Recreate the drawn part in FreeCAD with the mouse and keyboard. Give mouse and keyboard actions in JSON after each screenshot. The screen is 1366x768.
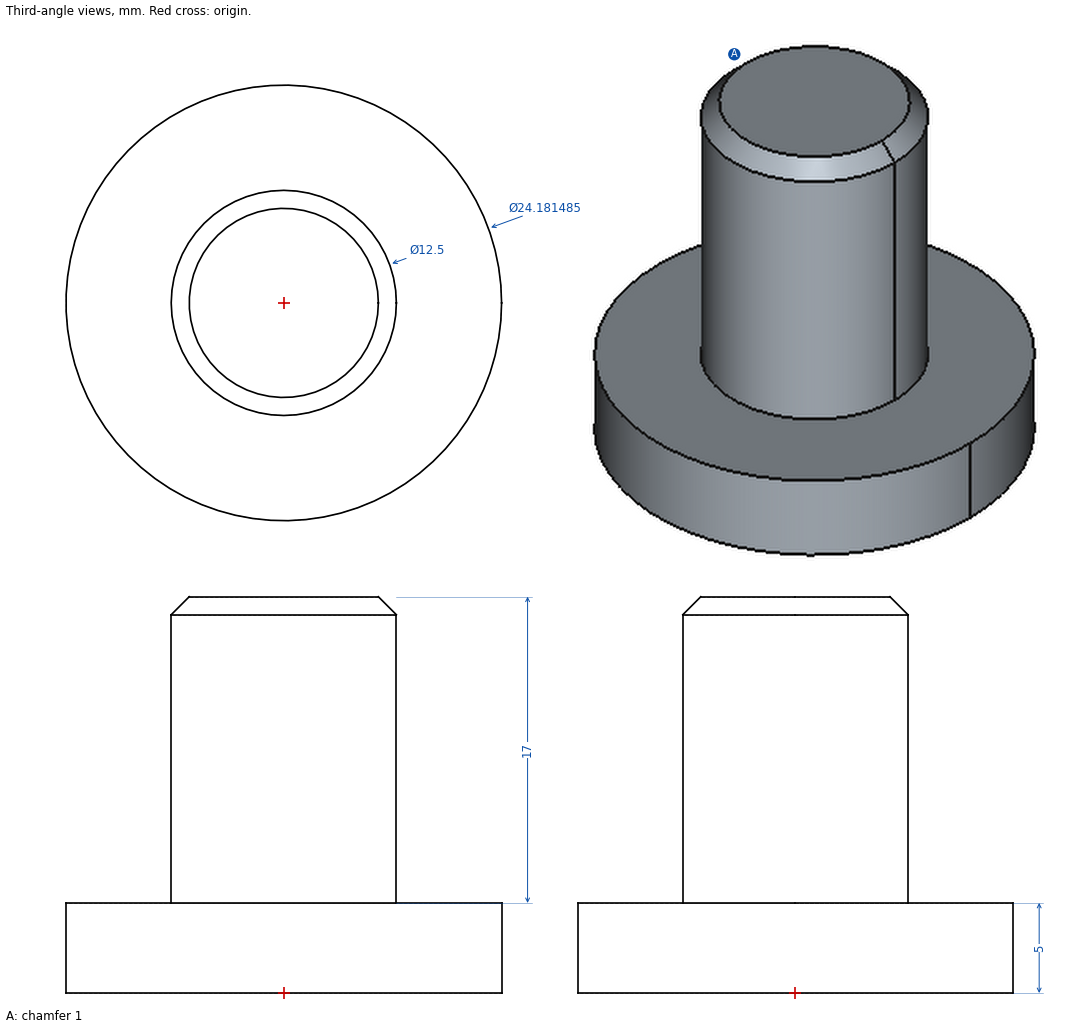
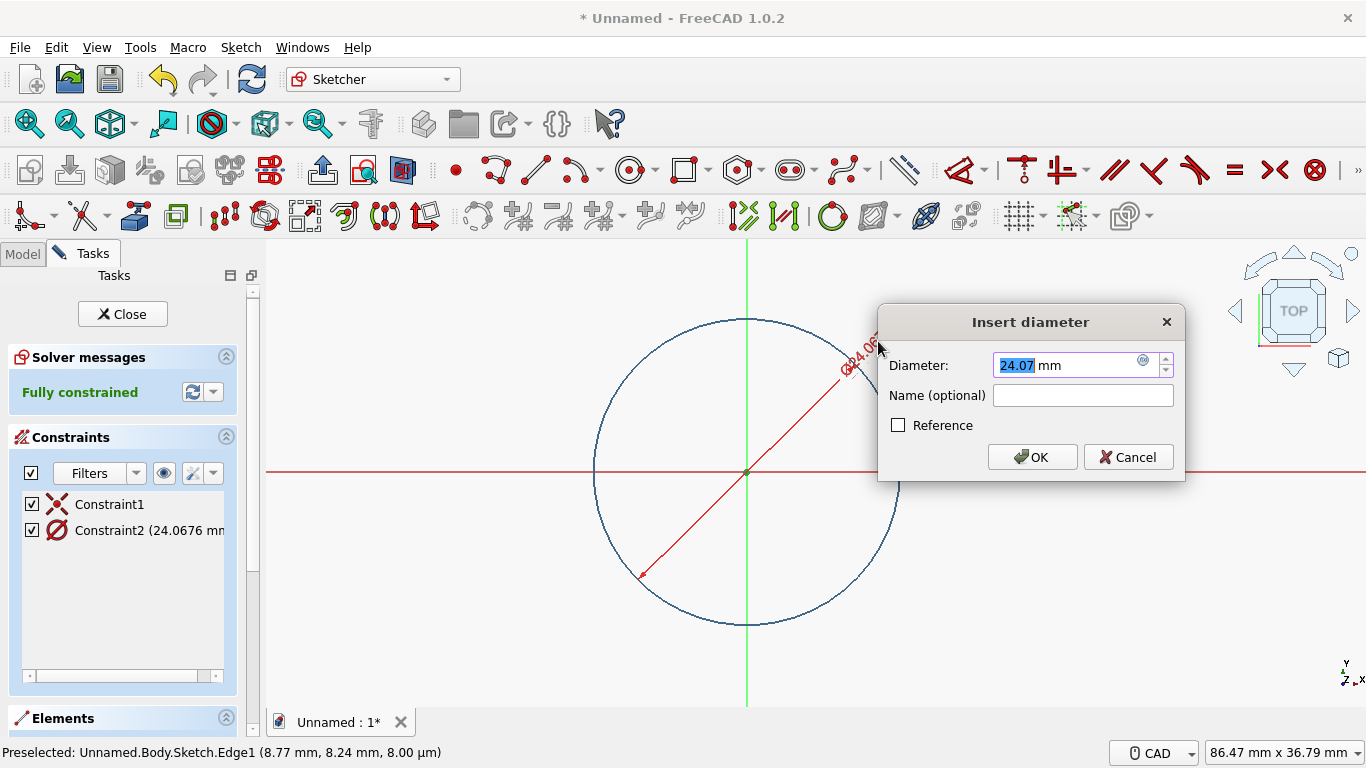
{"action": "type", "text": "24.181485"}
{"action": "key", "text": "Return"}
{"action": "key", "text": "Escape"}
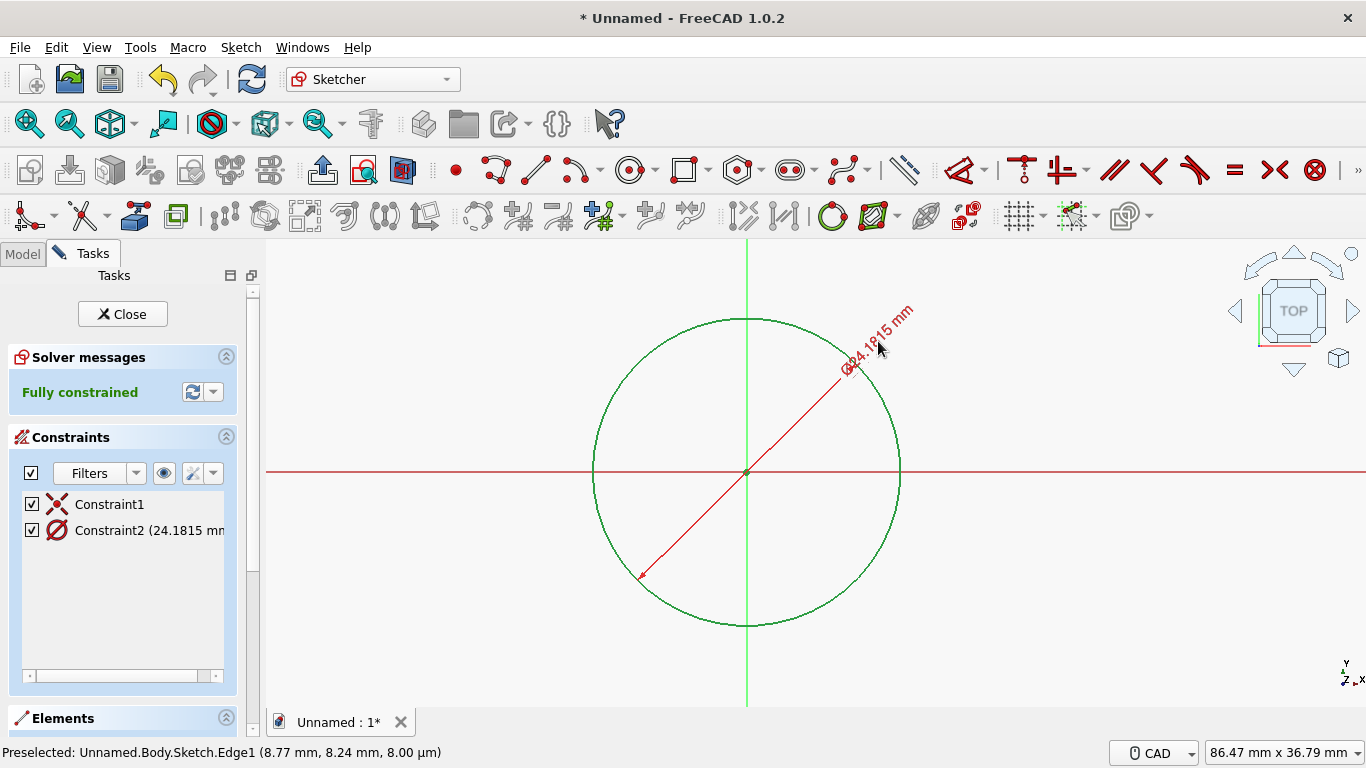
{"action": "left_click", "coordinate": [123, 314]}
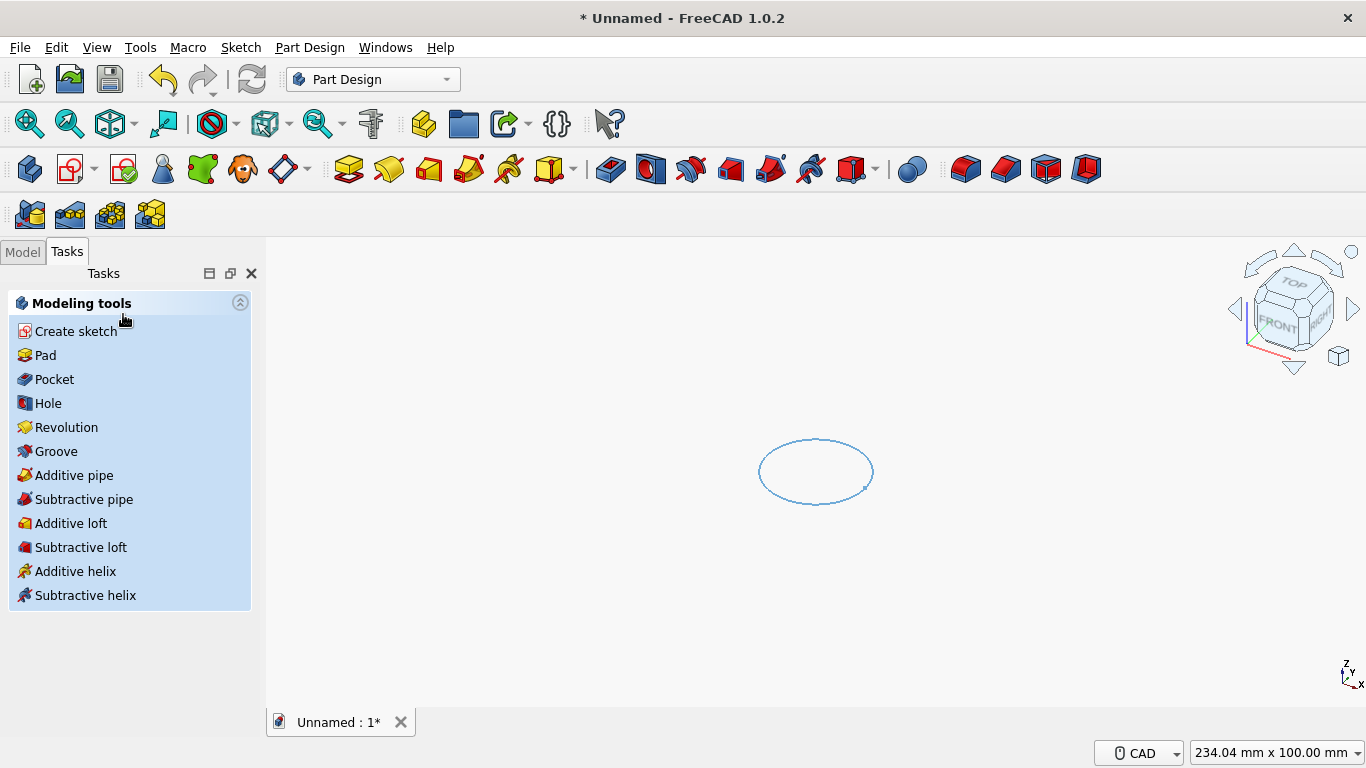
{"action": "left_click", "coordinate": [350, 170]}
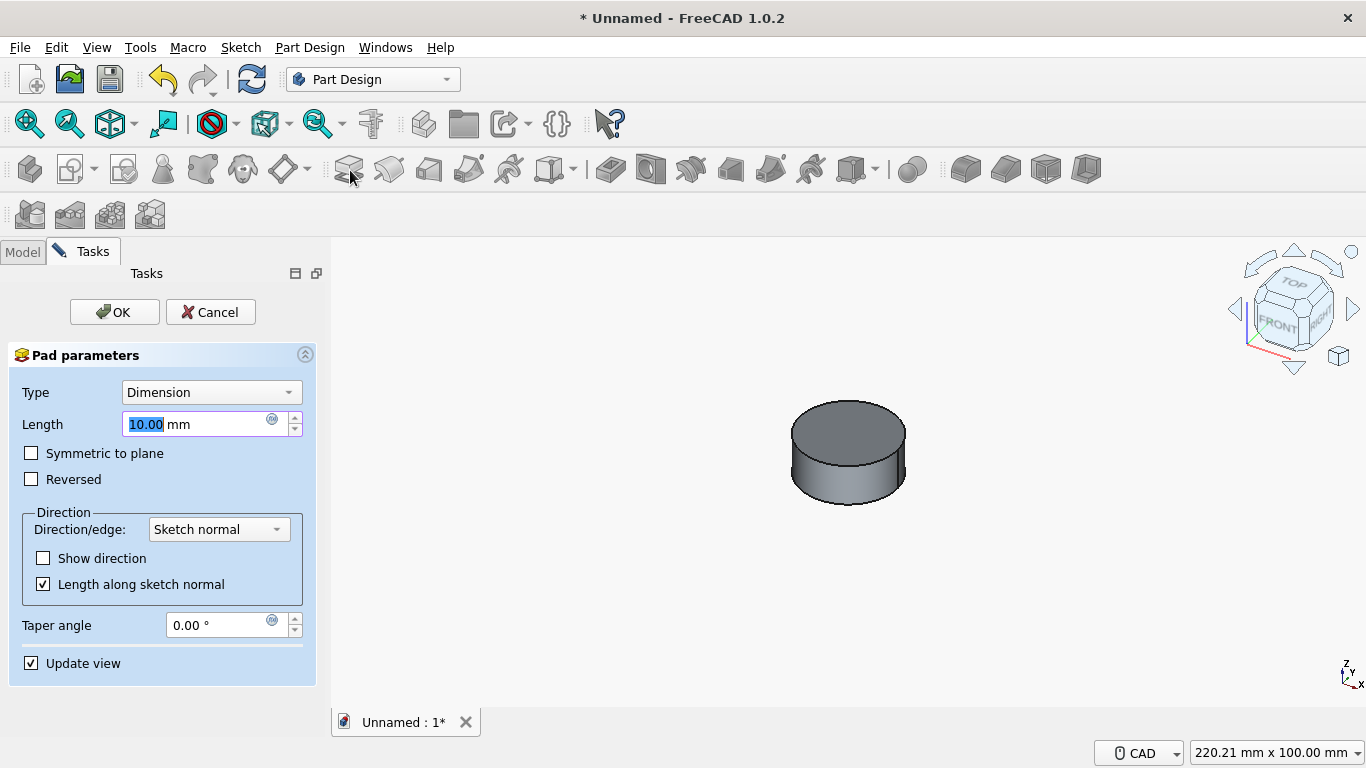
{"action": "type", "text": "5"}
{"action": "key", "text": "Tab"}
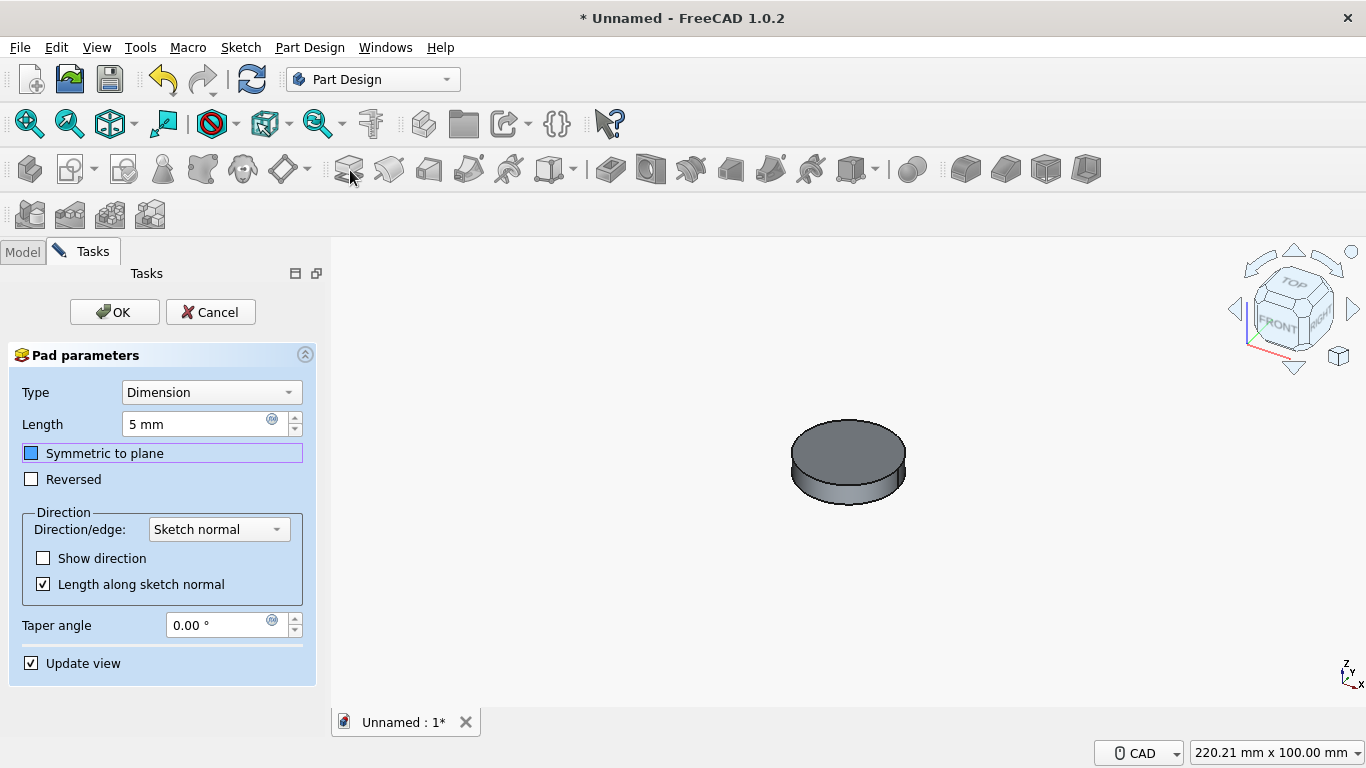
{"action": "left_click", "coordinate": [115, 312]}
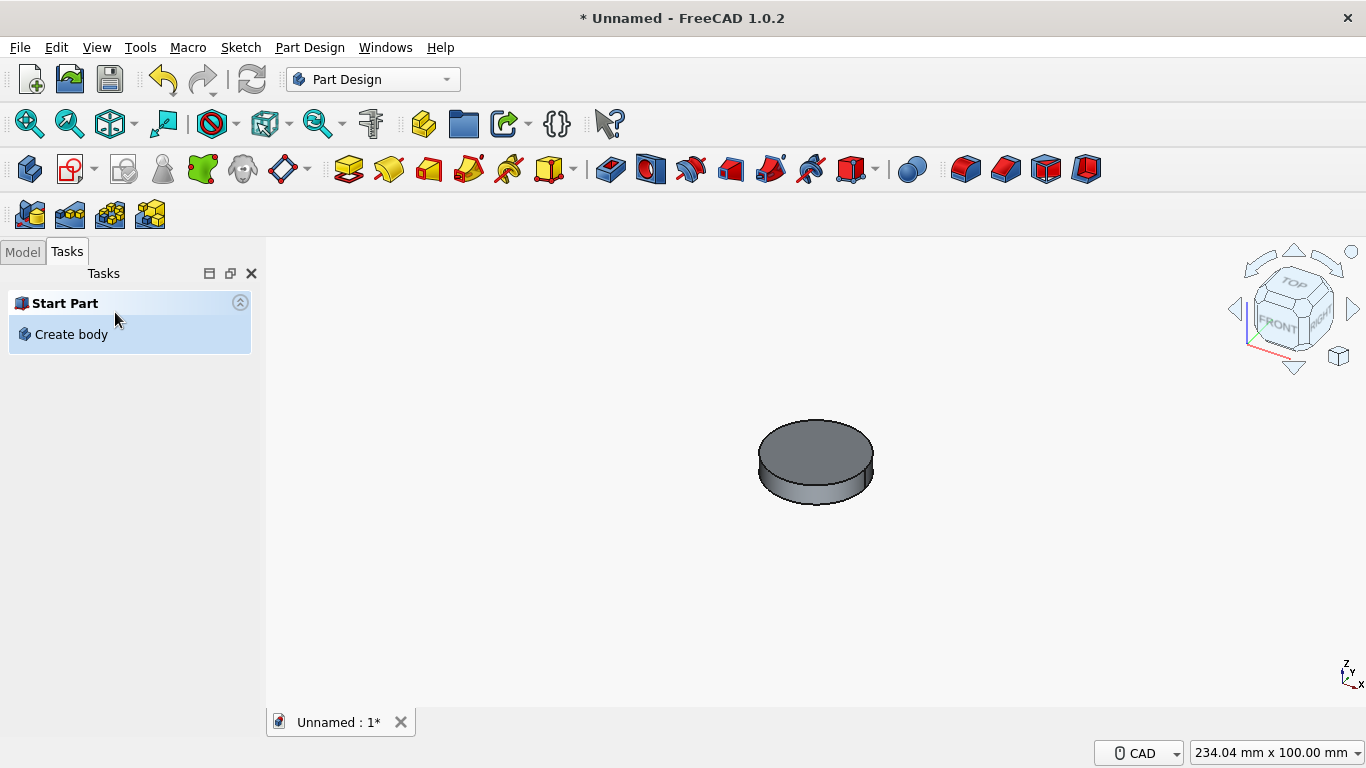
{"action": "left_click", "coordinate": [30, 124]}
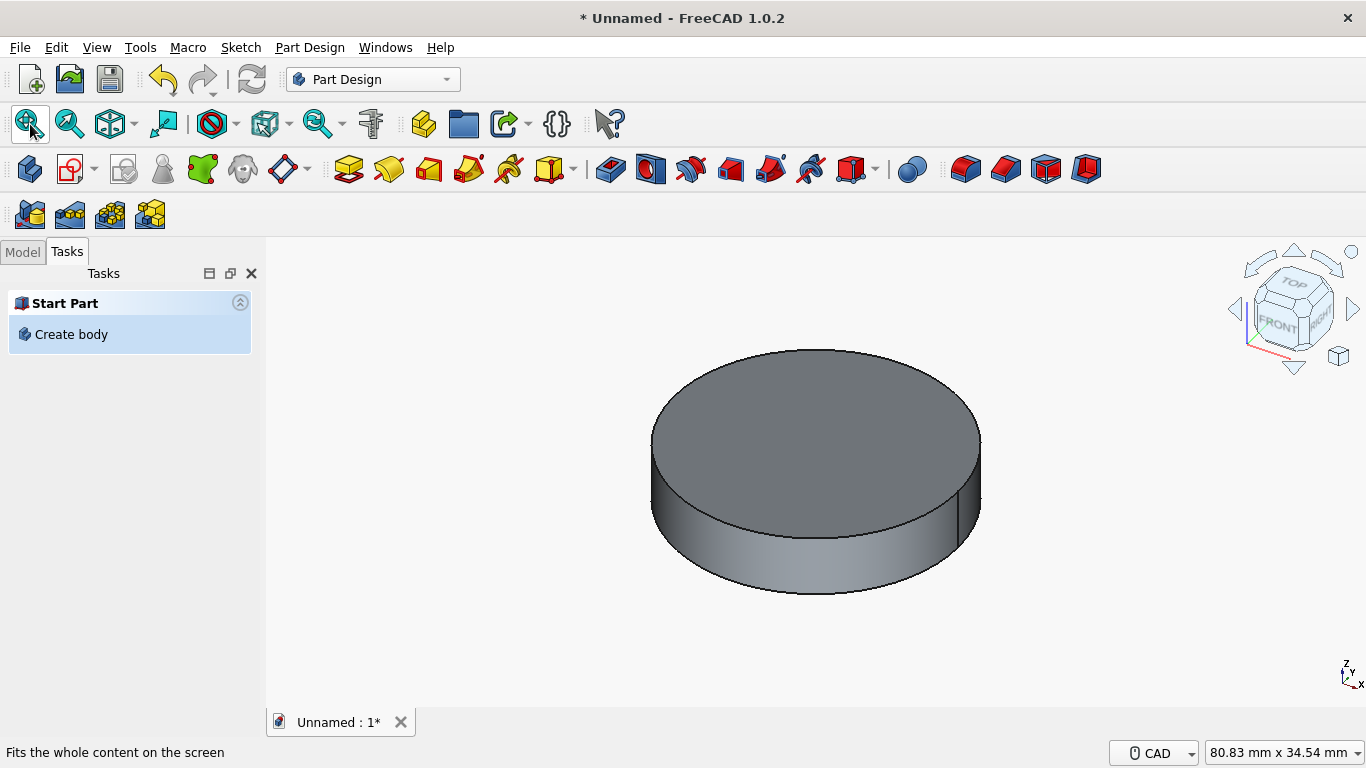
{"action": "left_click", "coordinate": [816, 443]}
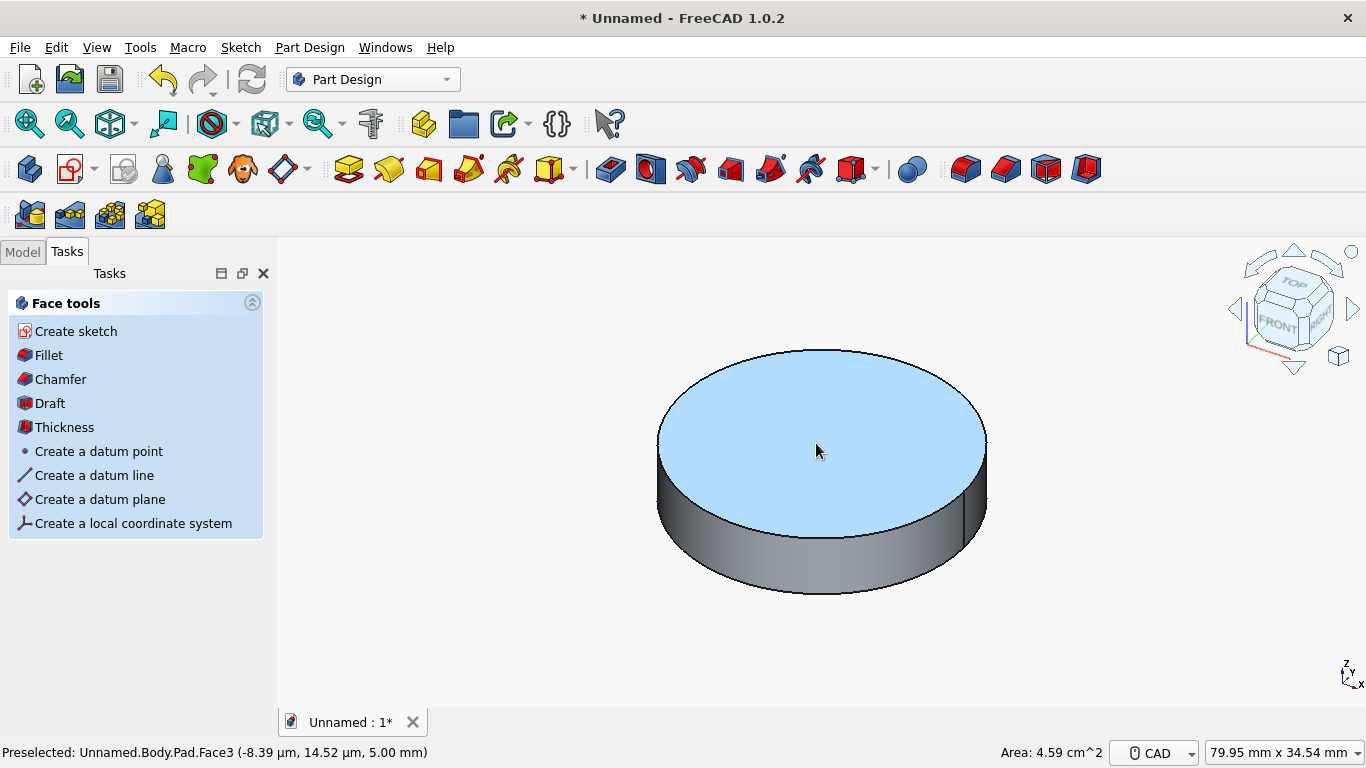
{"action": "left_click", "coordinate": [70, 170]}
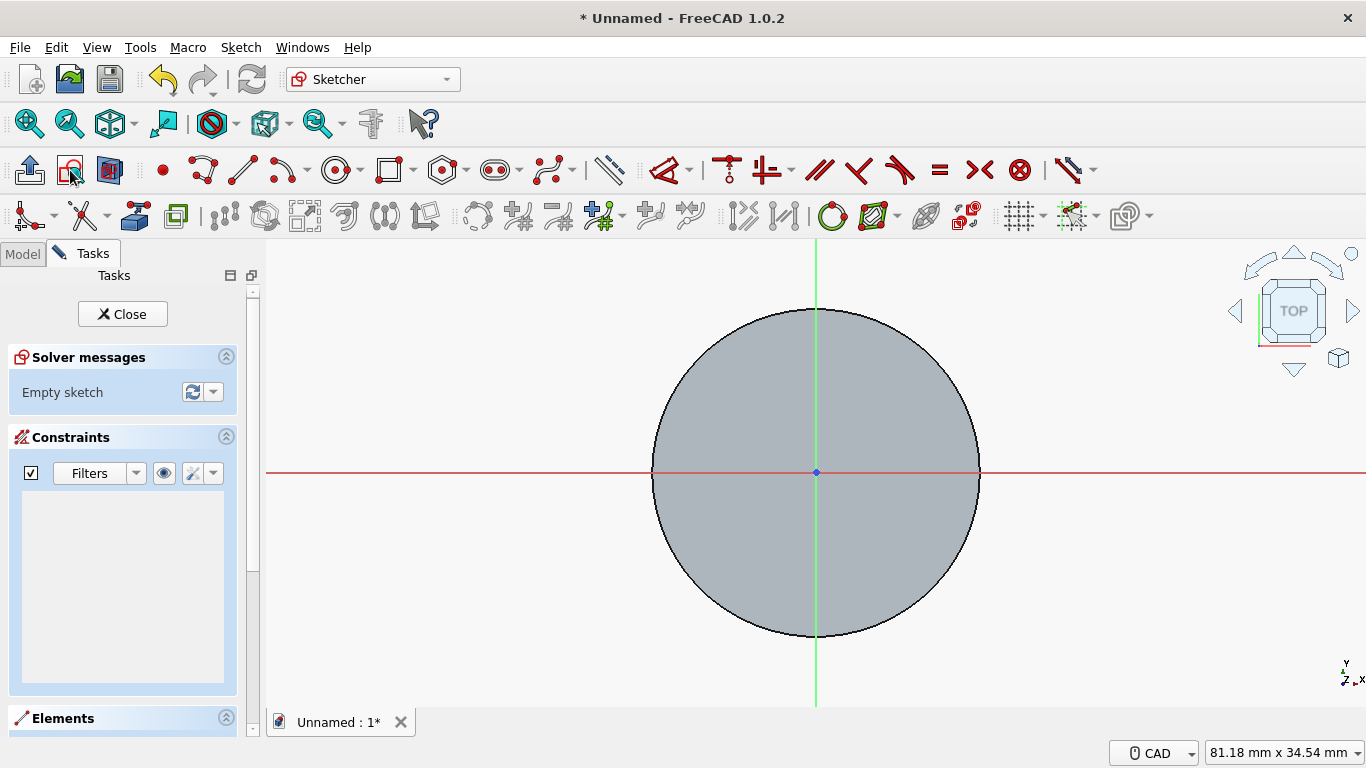
{"action": "scroll", "coordinate": [899, 473], "scroll_direction": "up", "scroll_amount": 3}